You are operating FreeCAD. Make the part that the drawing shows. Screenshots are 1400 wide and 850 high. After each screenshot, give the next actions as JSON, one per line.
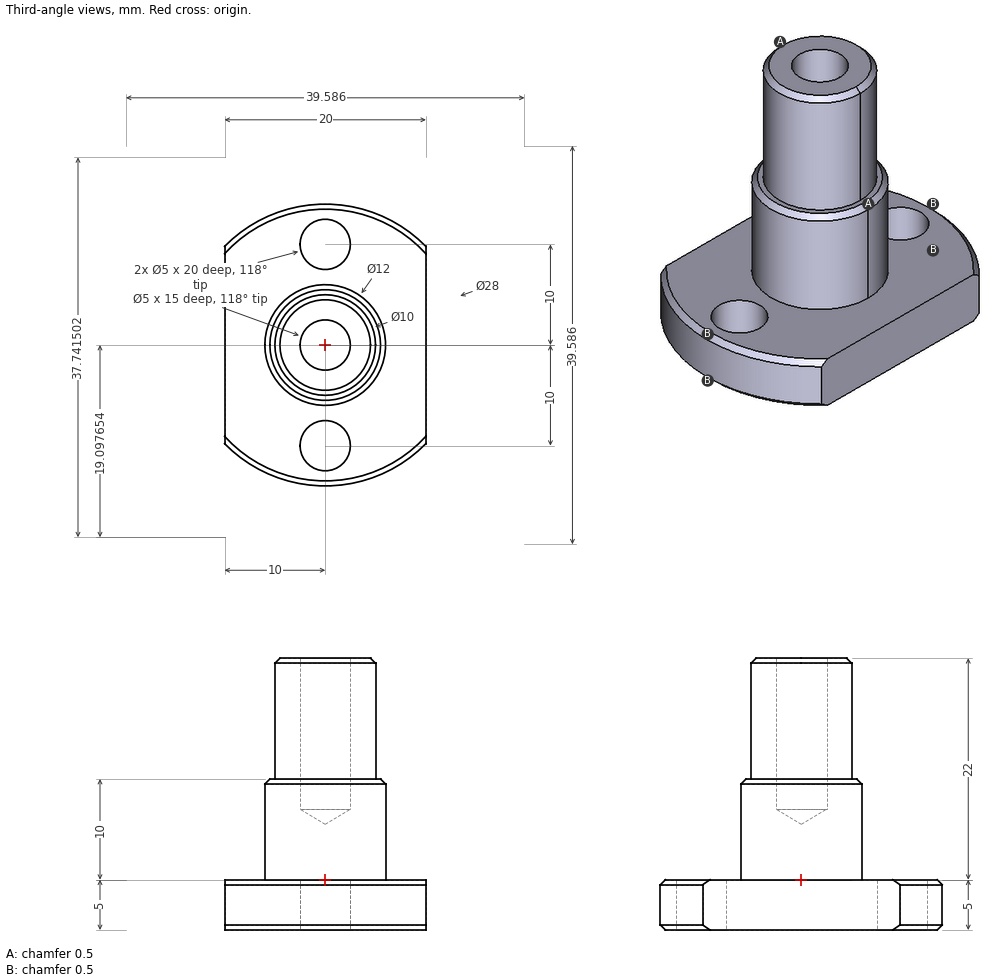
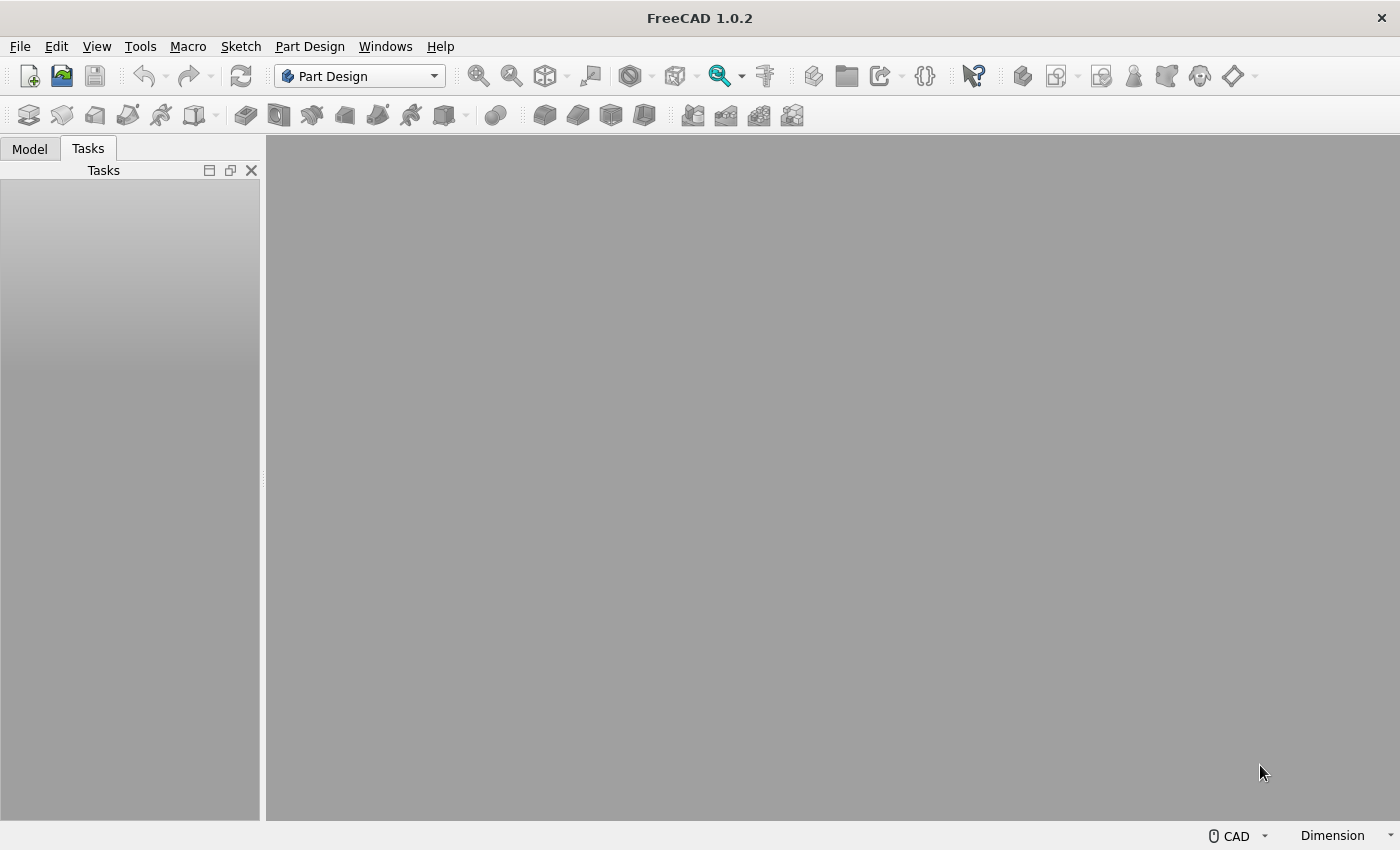
{"action": "key", "text": "ctrl+n"}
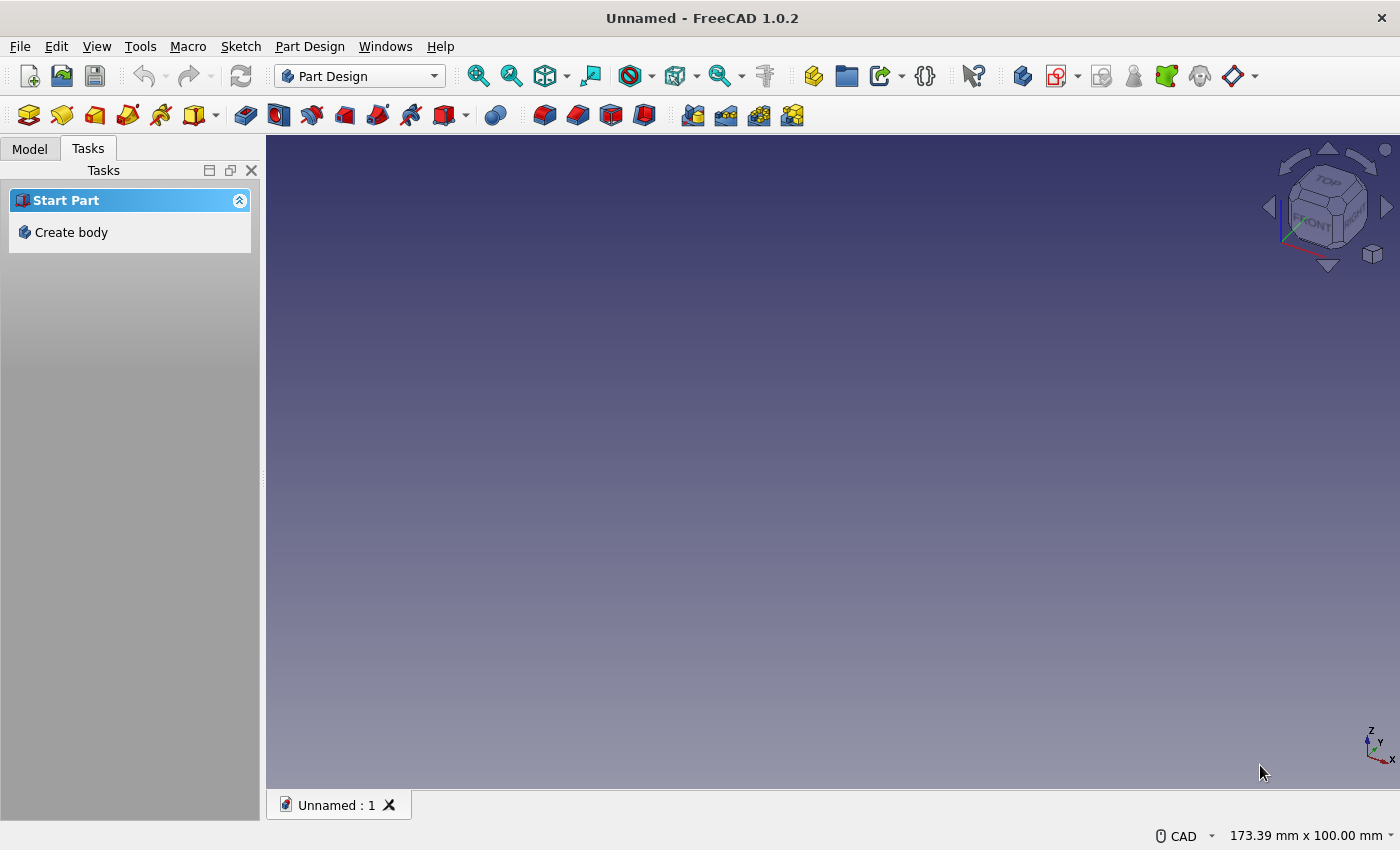
{"action": "left_click", "coordinate": [1056, 76]}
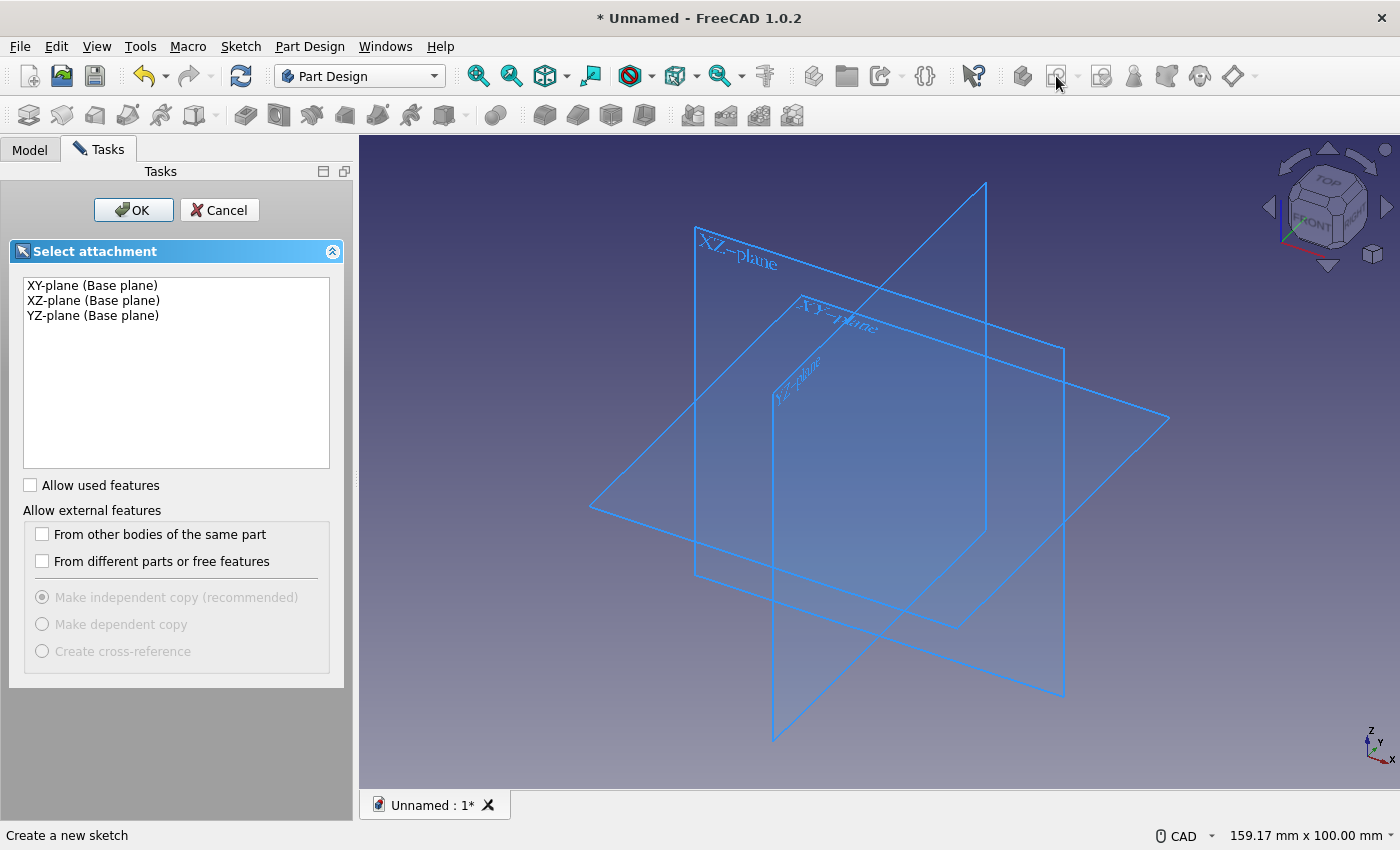
{"action": "left_click", "coordinate": [84, 286]}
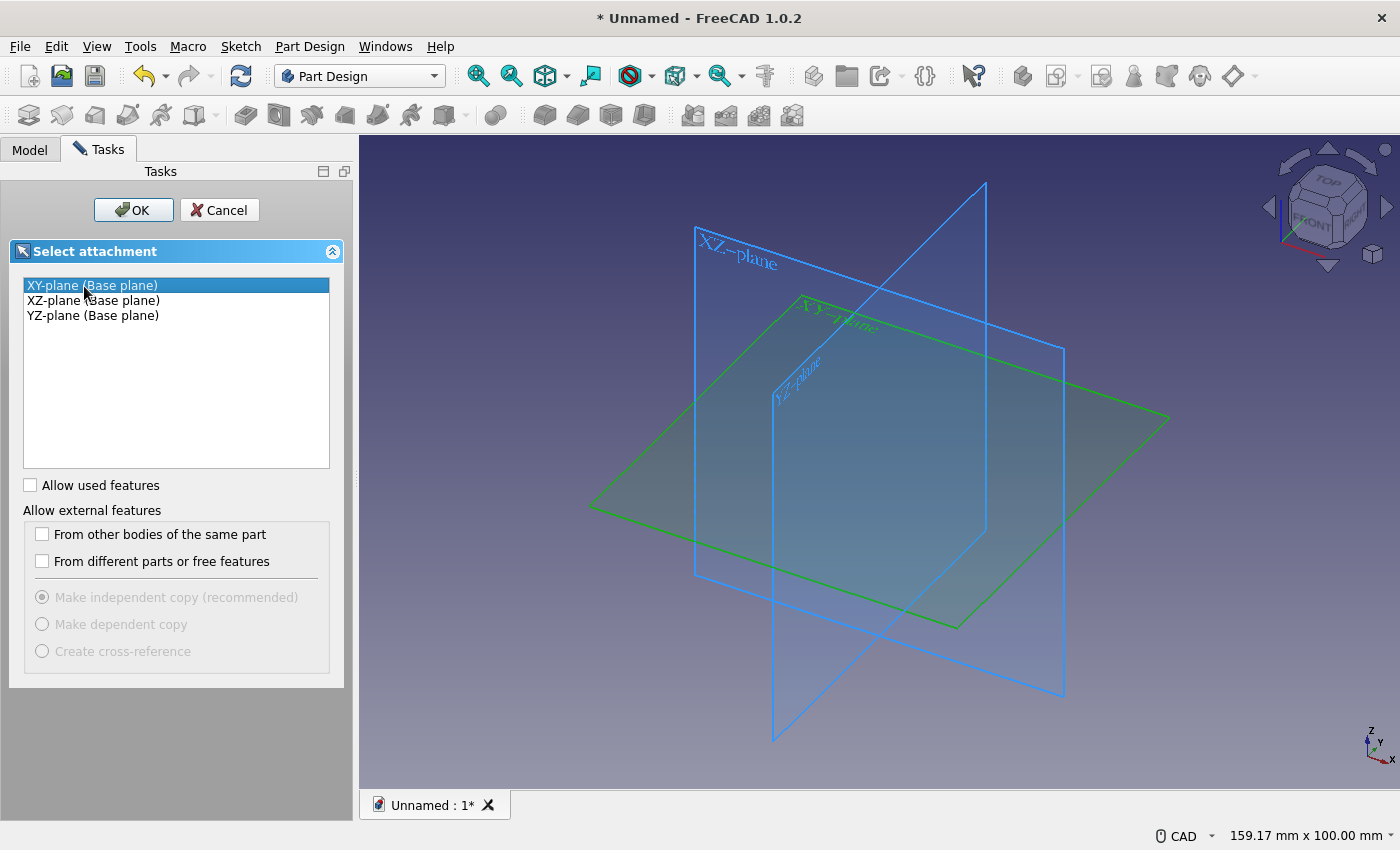
{"action": "left_click", "coordinate": [134, 210]}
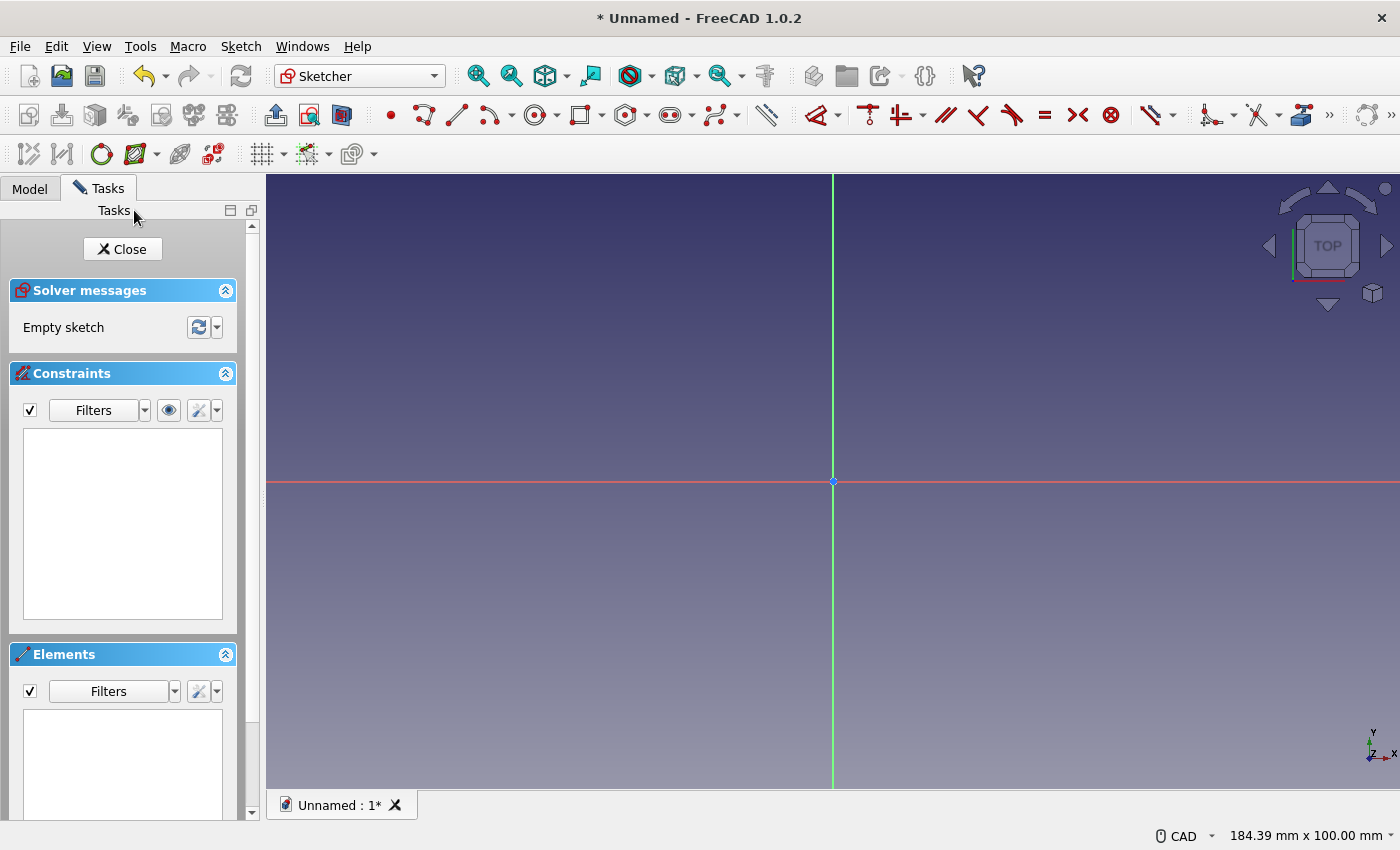
{"action": "scroll", "coordinate": [847, 482], "scroll_direction": "up", "scroll_amount": 9}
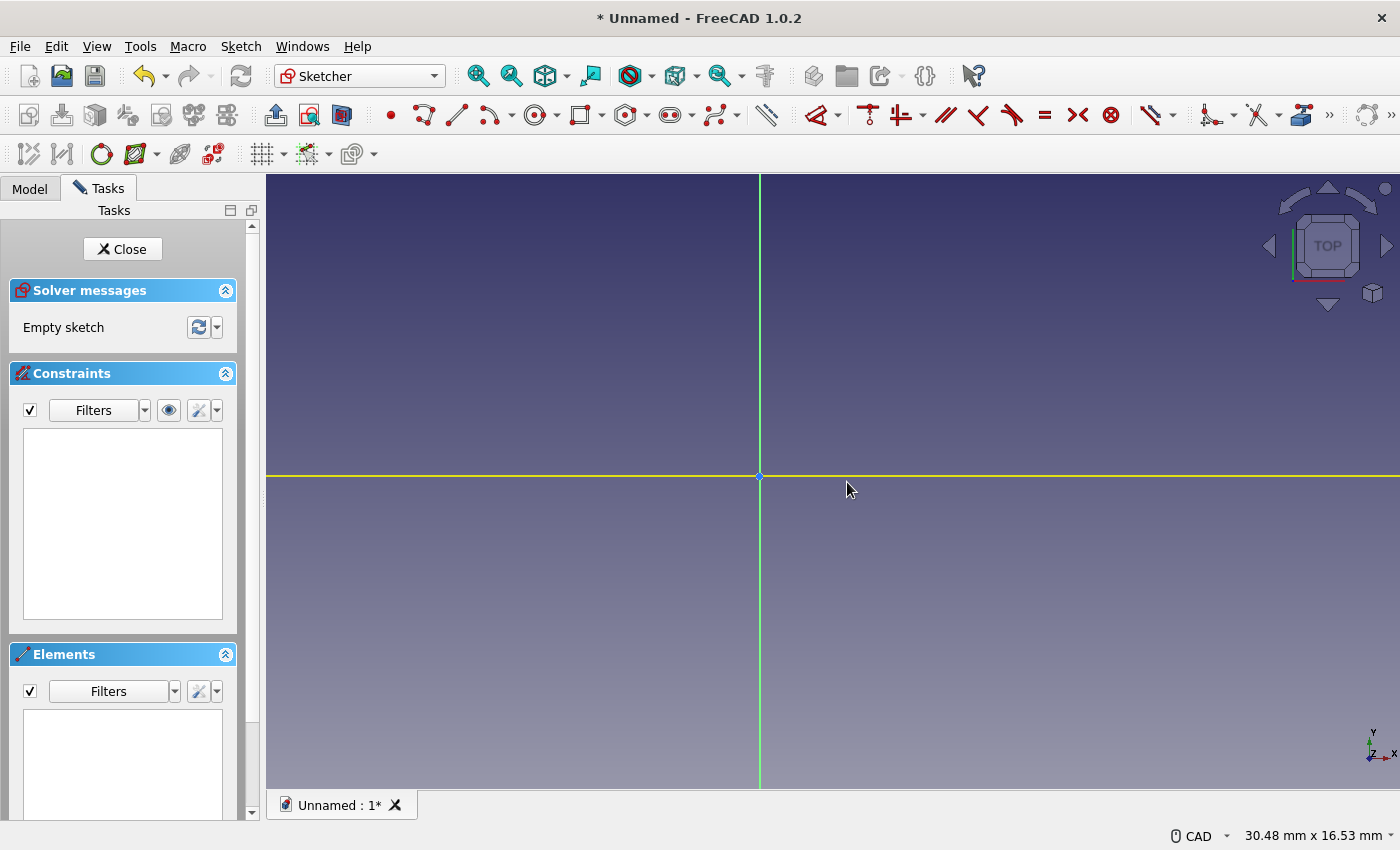
{"action": "key", "text": "g c"}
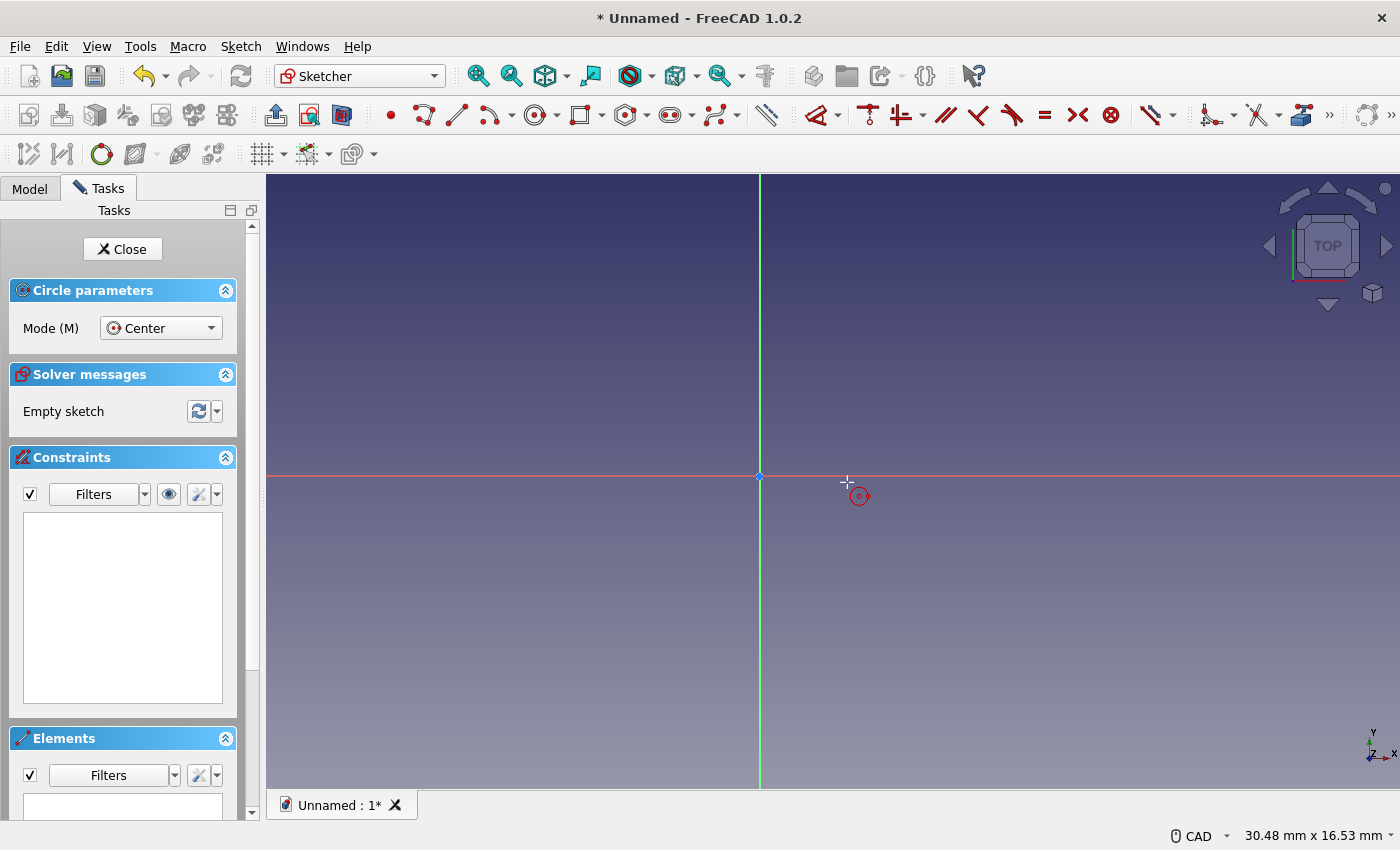
{"action": "left_click", "coordinate": [760, 476]}
{"action": "mouse_move", "coordinate": [891, 345]}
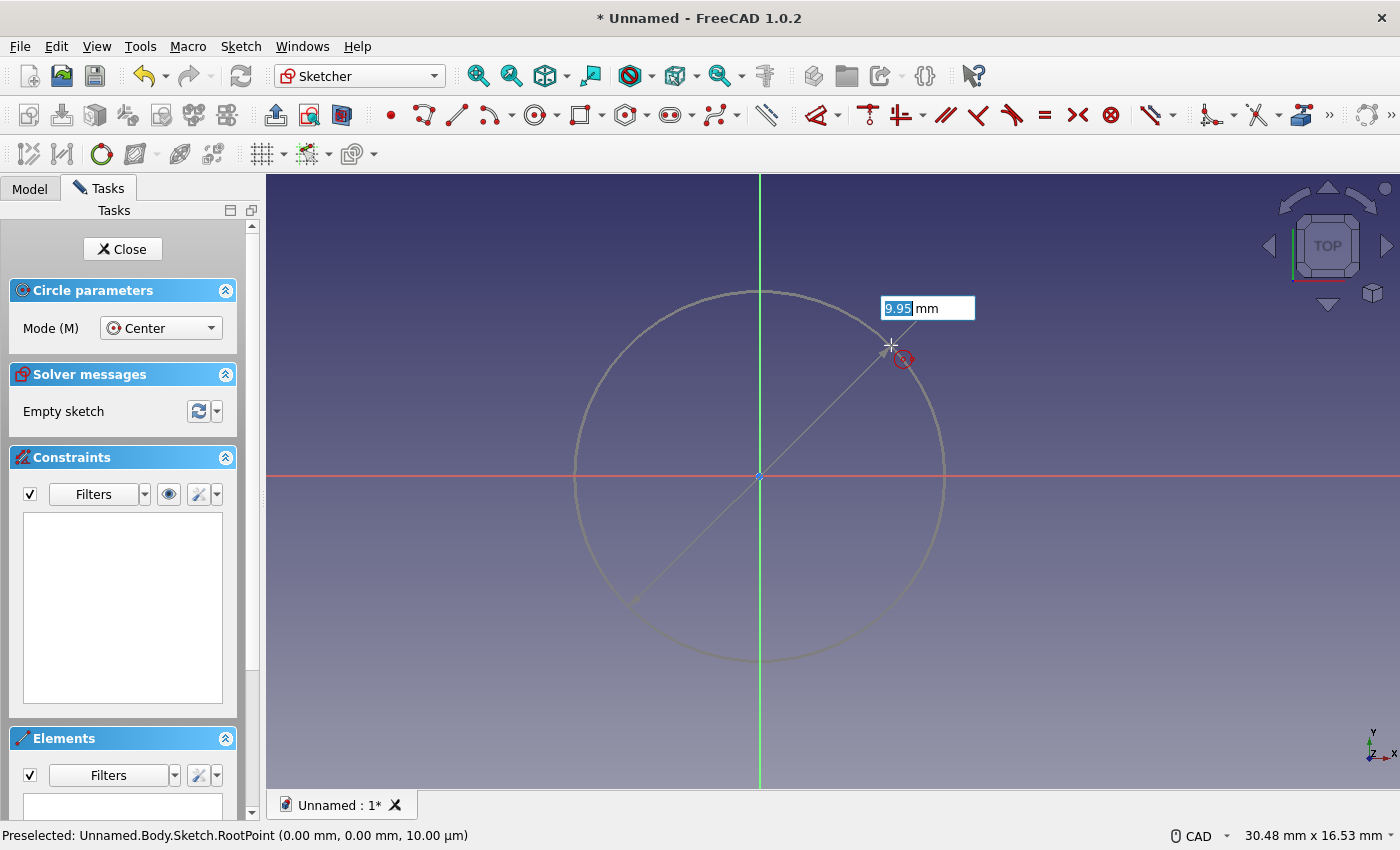
{"action": "type", "text": "10"}
{"action": "key", "text": "Return"}
{"action": "key", "text": "Escape"}